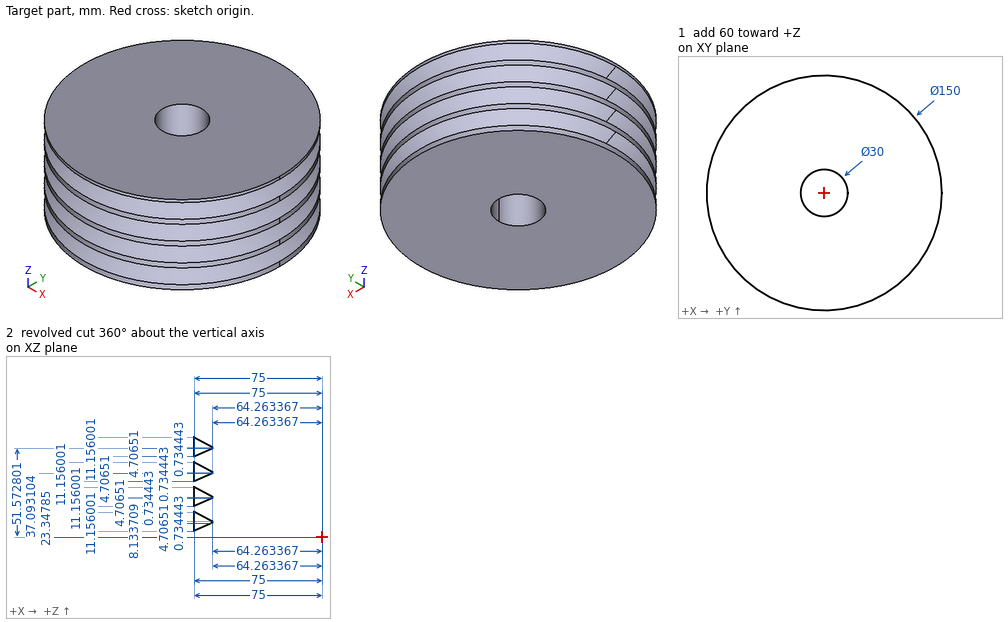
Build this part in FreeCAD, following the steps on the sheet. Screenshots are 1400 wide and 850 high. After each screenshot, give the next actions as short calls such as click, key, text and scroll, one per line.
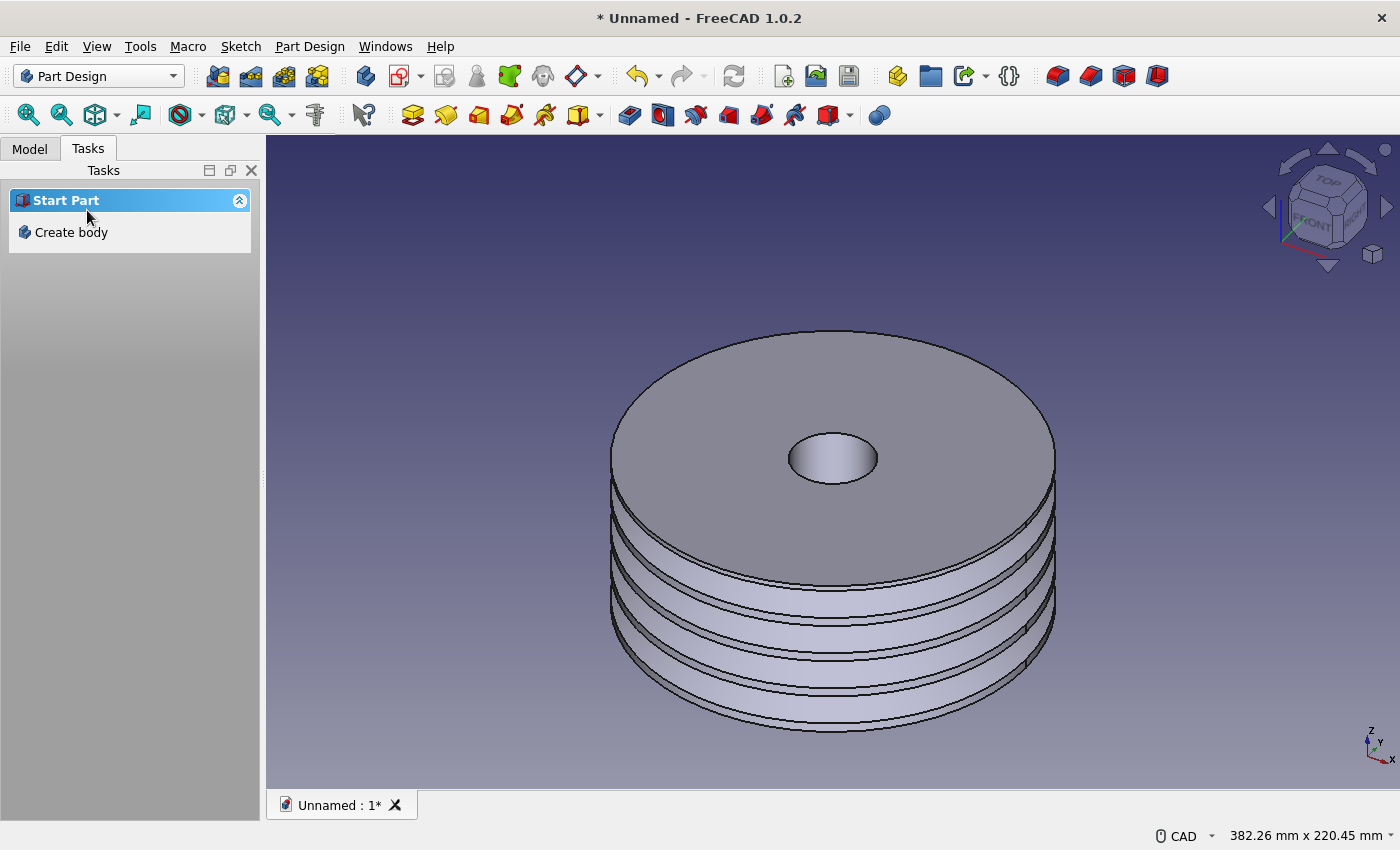
key(0)